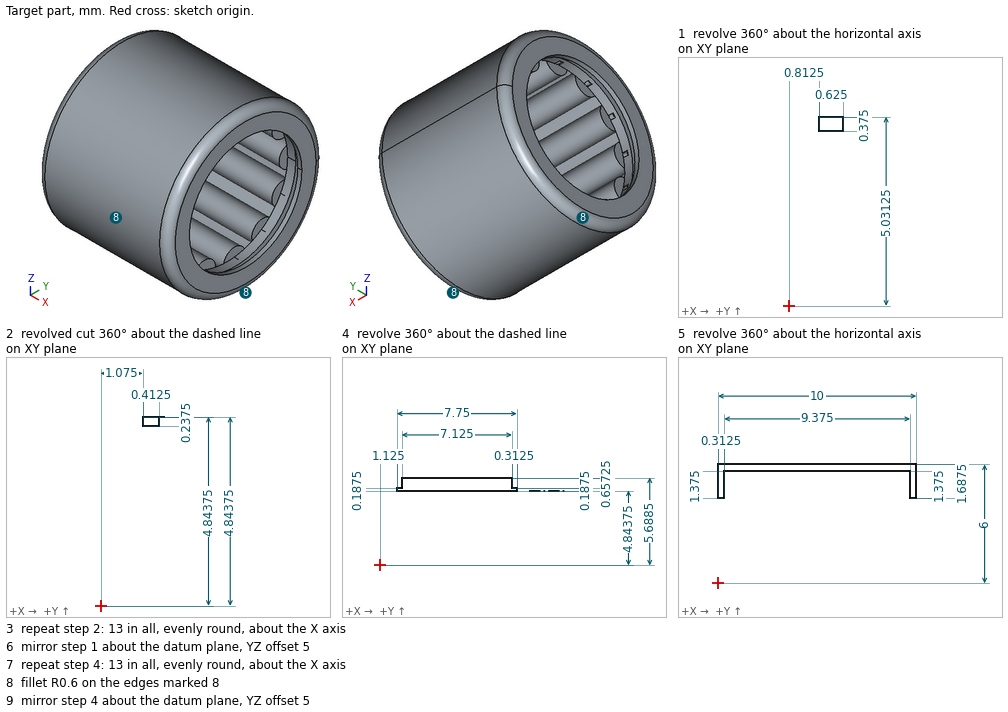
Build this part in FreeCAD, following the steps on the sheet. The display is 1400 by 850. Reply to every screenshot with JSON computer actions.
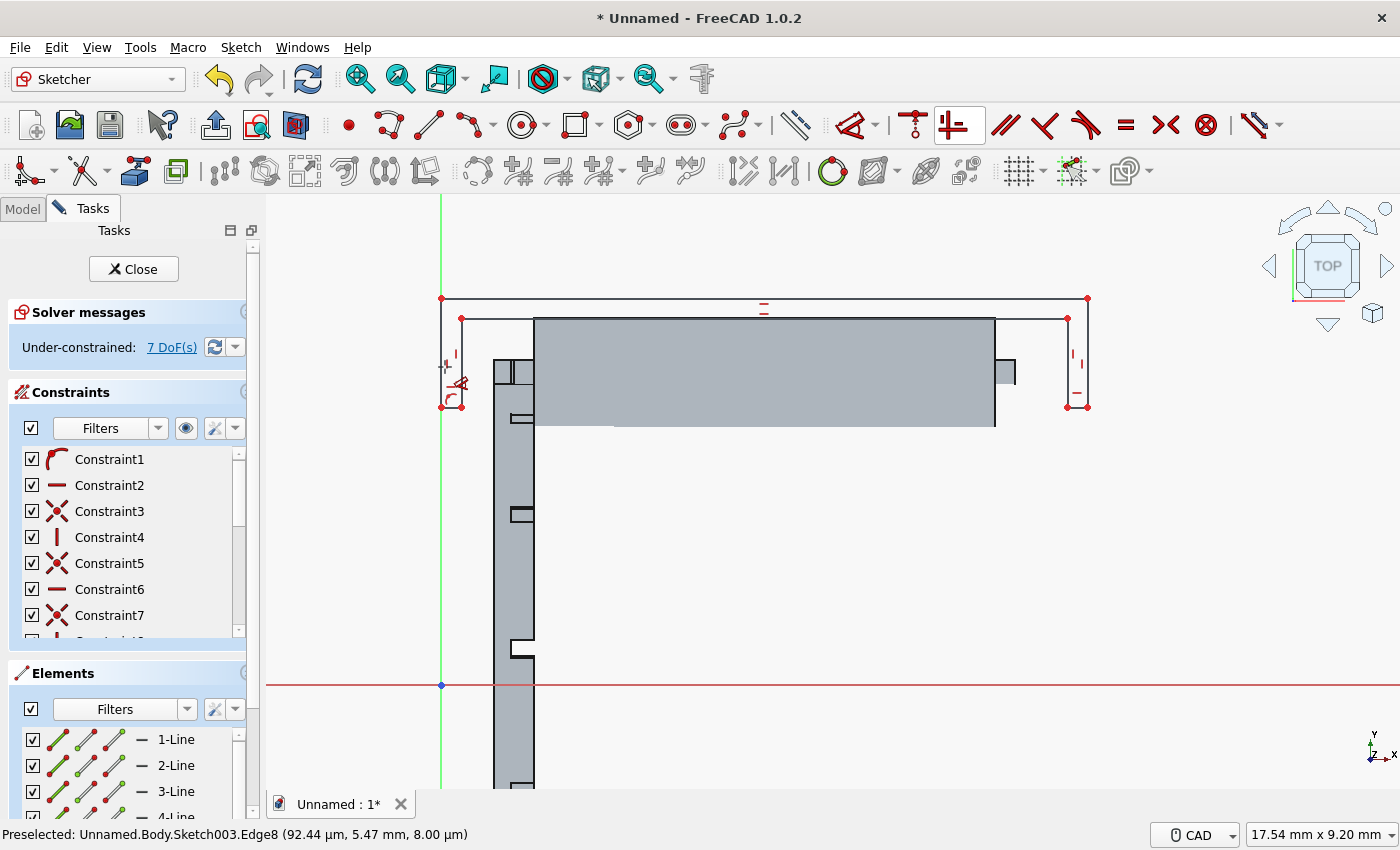
{"action": "left_click", "coordinate": [894, 299]}
{"action": "left_click", "coordinate": [765, 265]}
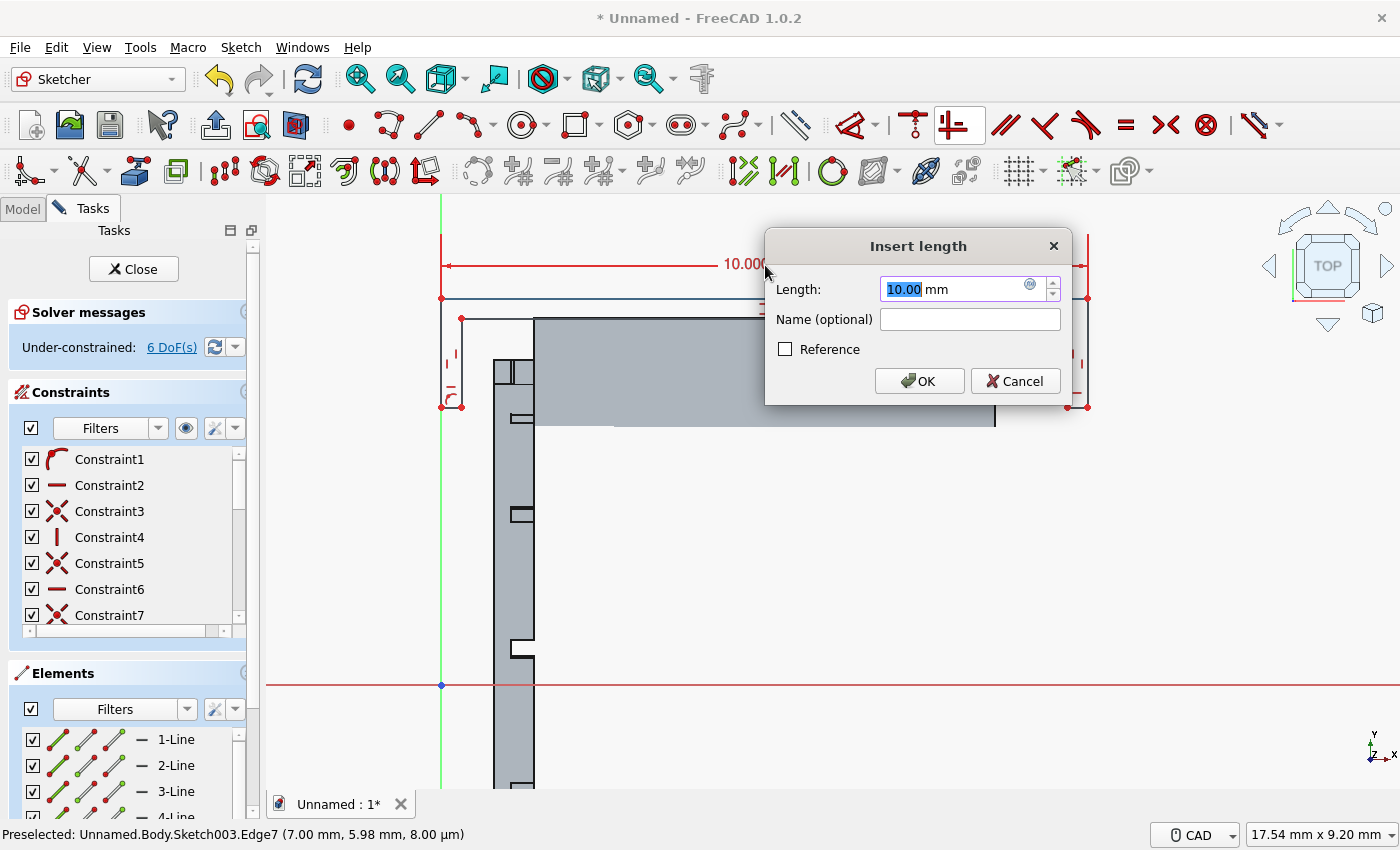
{"action": "type", "text": "10"}
{"action": "key", "text": "Return"}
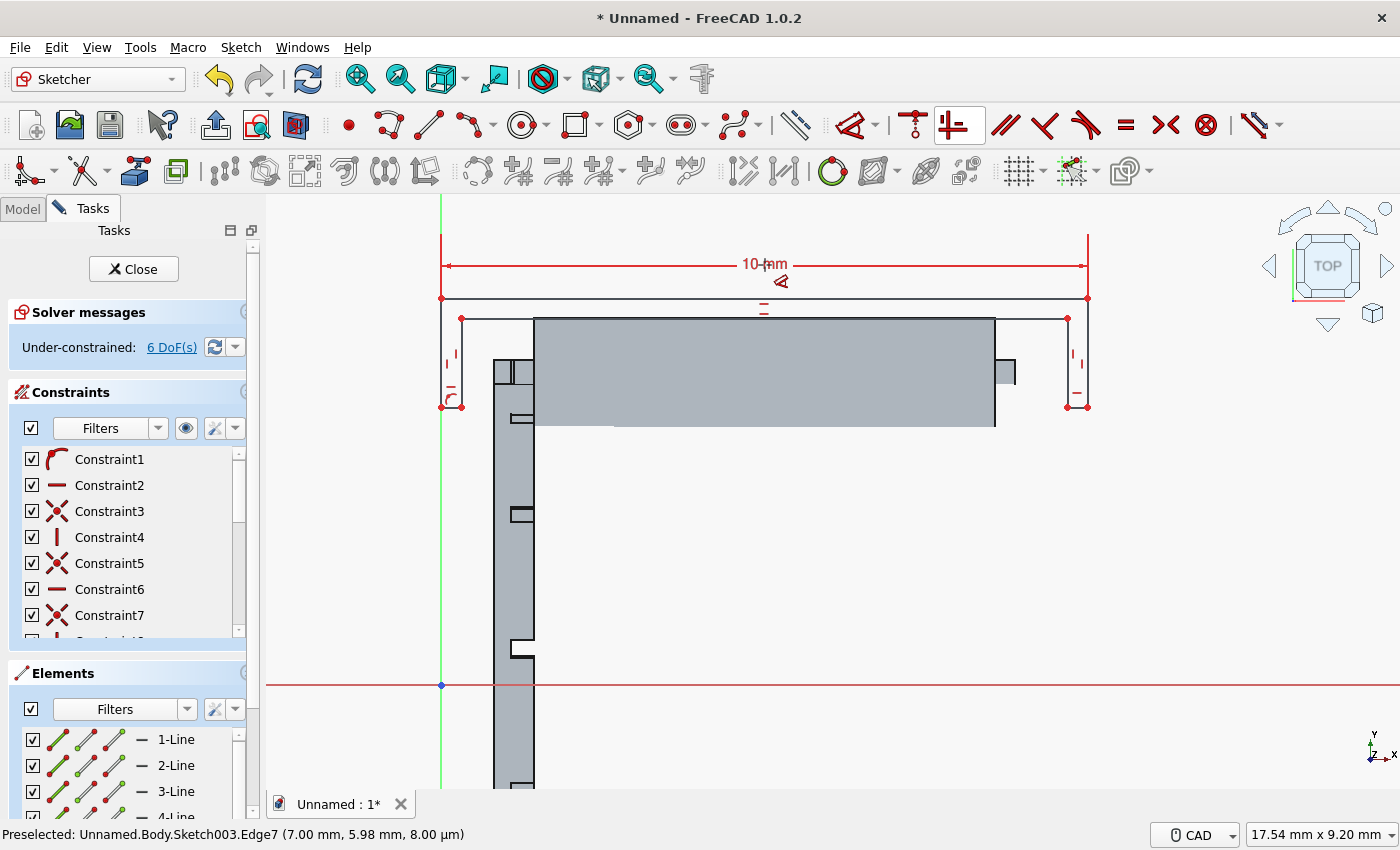
{"action": "left_click", "coordinate": [1088, 299]}
{"action": "left_click", "coordinate": [407, 492]}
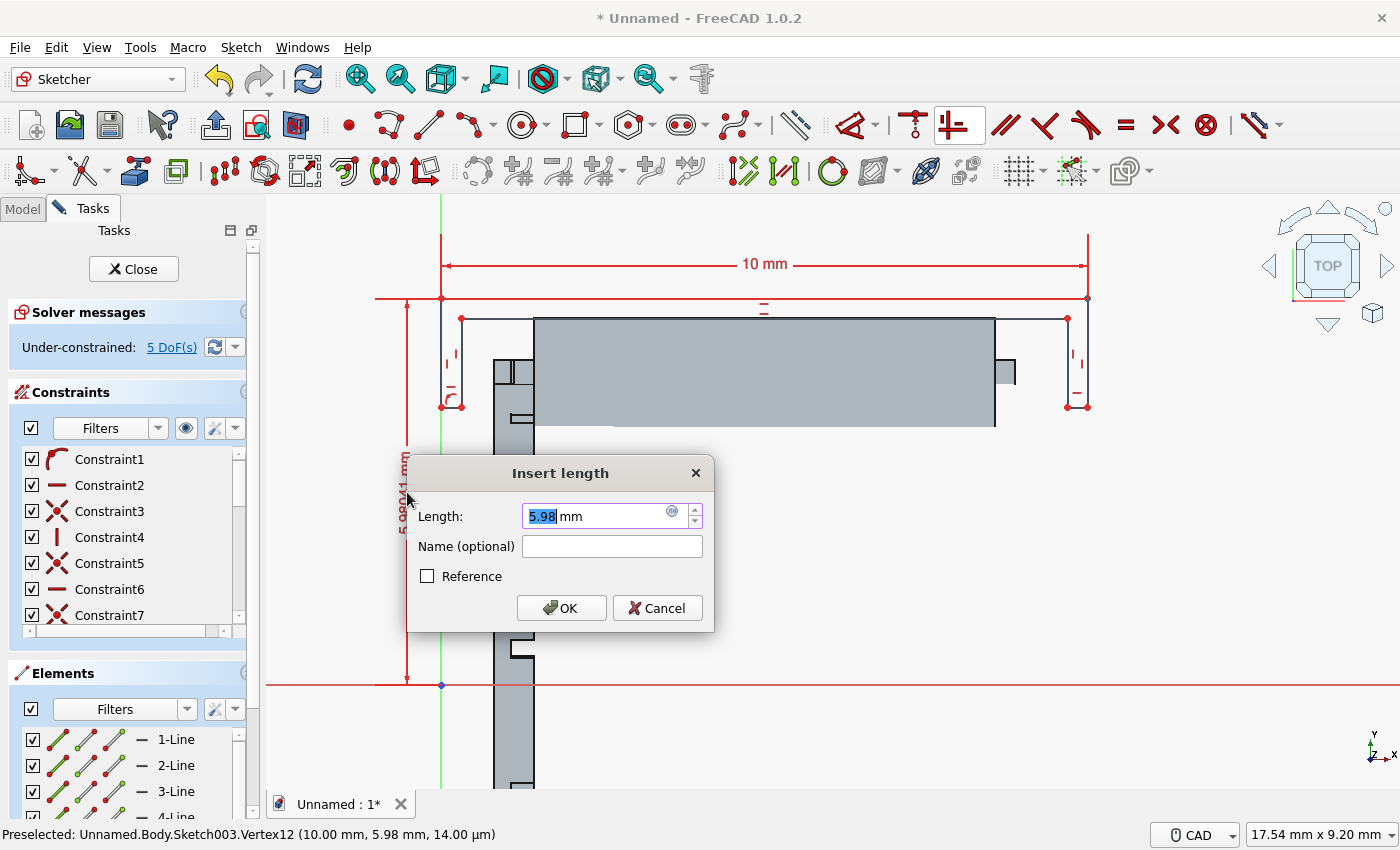
{"action": "type", "text": "6"}
{"action": "key", "text": "Return"}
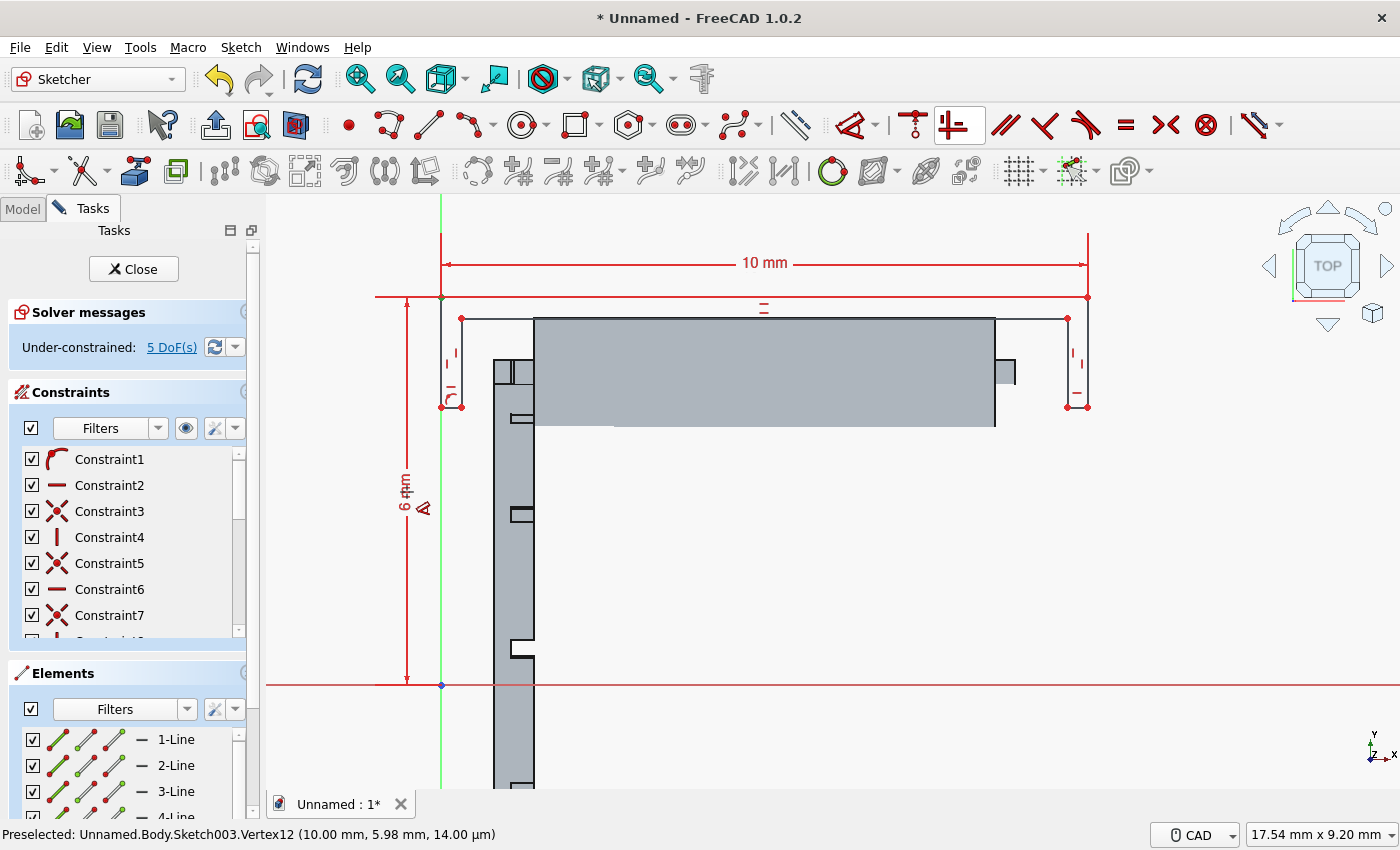
{"action": "left_click", "coordinate": [462, 381]}
{"action": "left_click", "coordinate": [428, 363]}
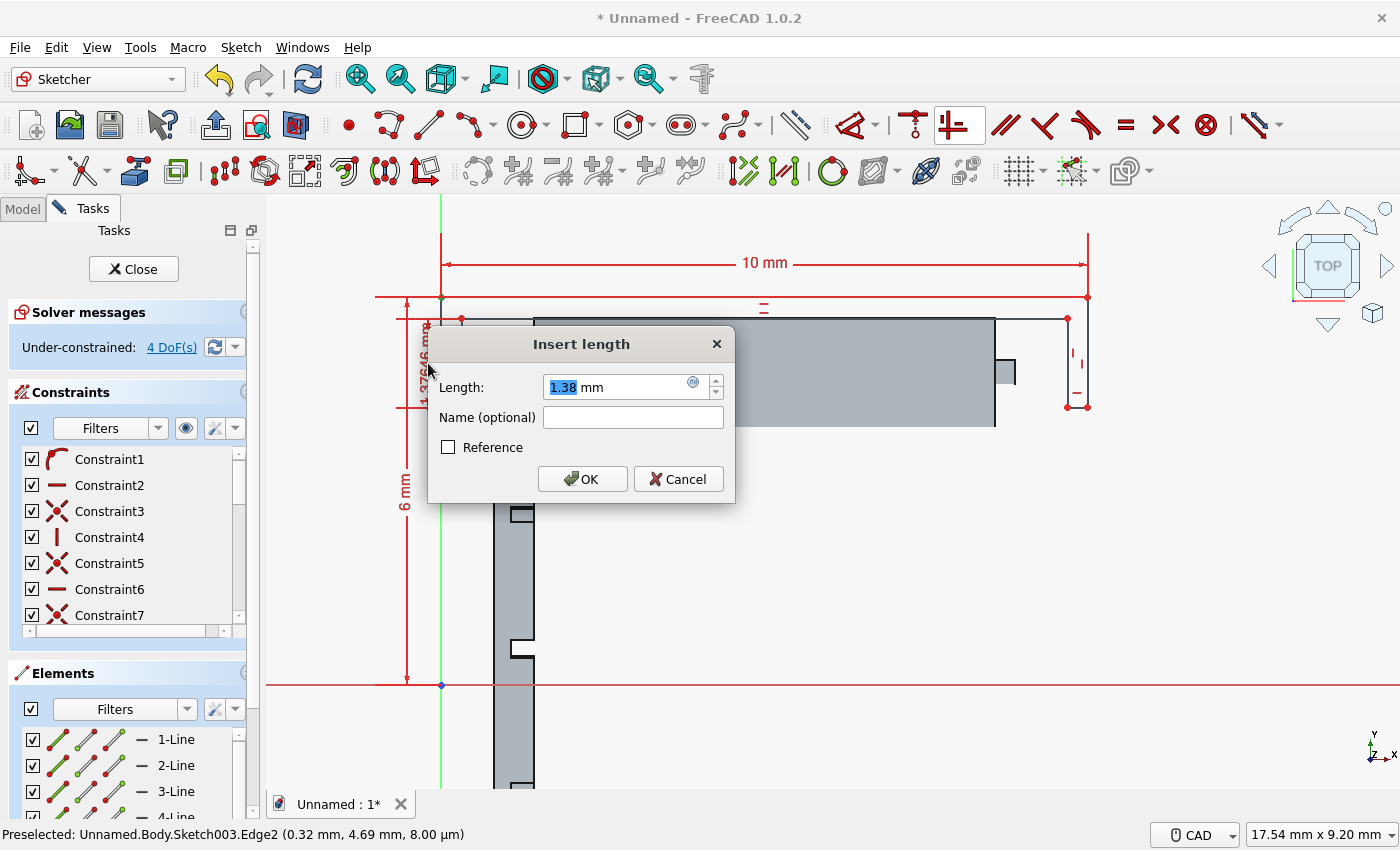
{"action": "type", "text": "1.375"}
{"action": "key", "text": "Return"}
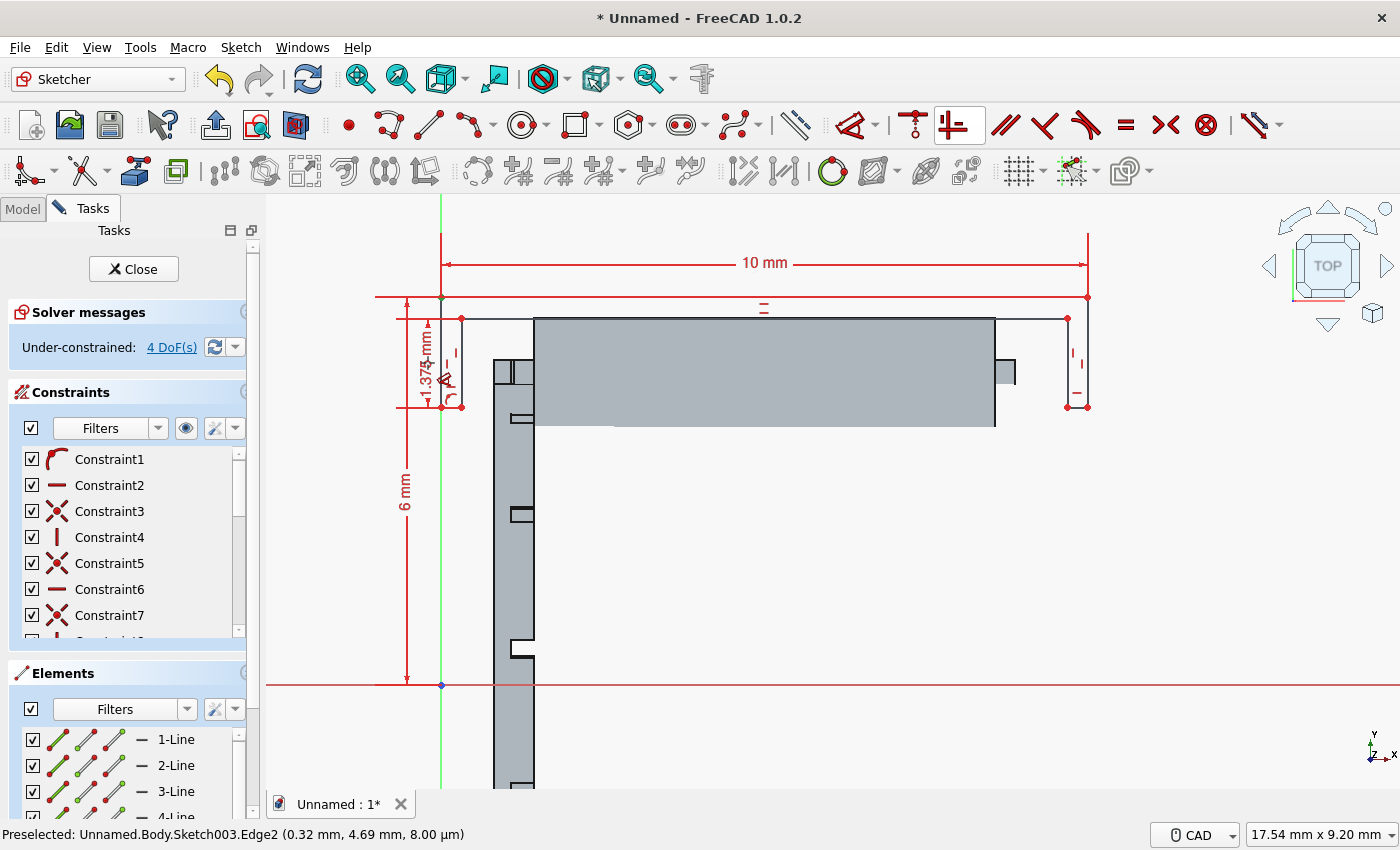
{"action": "left_click", "coordinate": [644, 319]}
{"action": "left_click", "coordinate": [765, 353]}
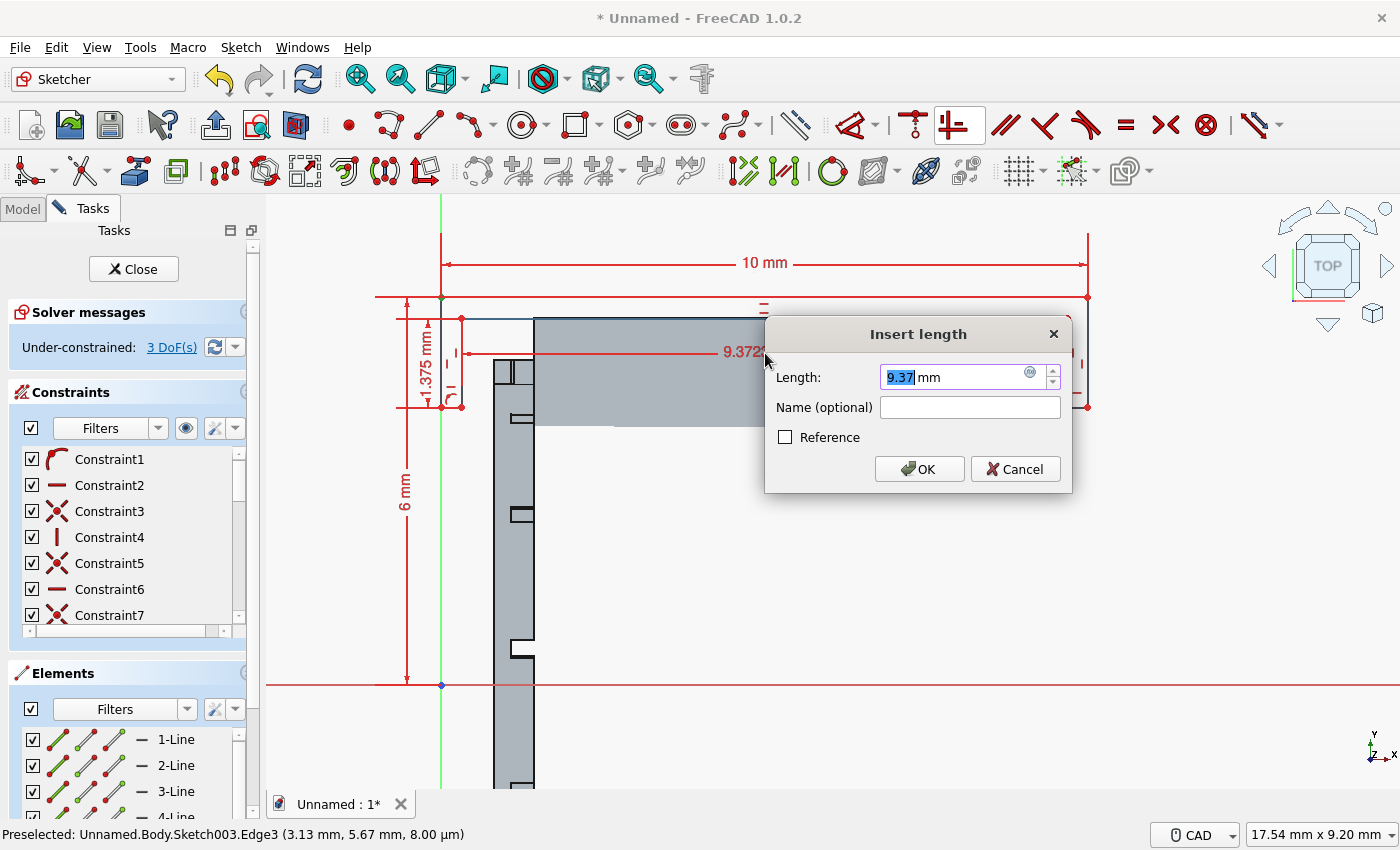
{"action": "type", "text": "9.375"}
{"action": "key", "text": "Return"}